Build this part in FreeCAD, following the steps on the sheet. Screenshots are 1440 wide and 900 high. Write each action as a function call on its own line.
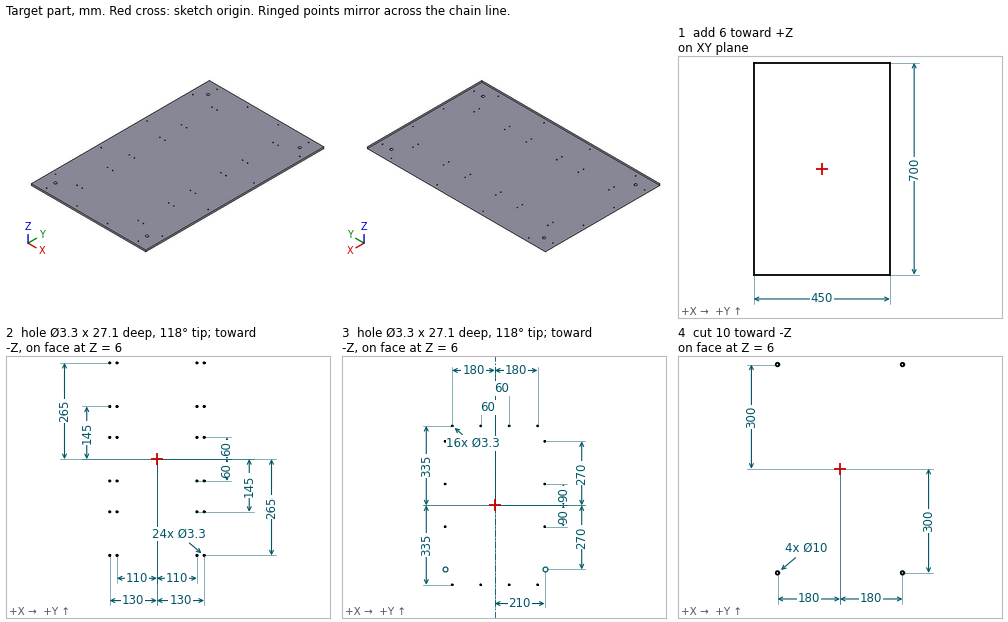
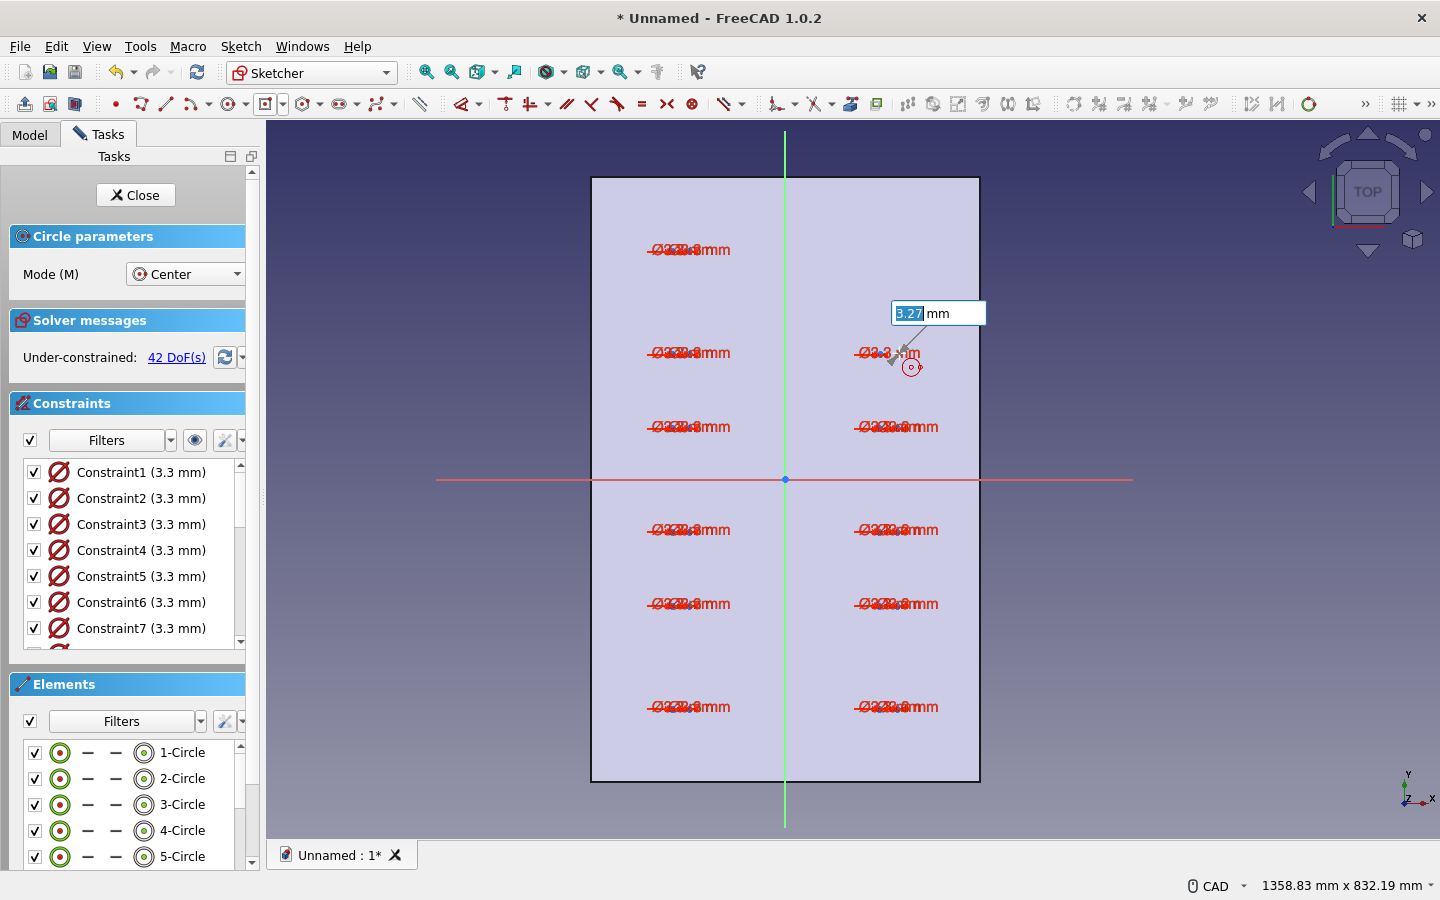
text(3.3)
key(Return)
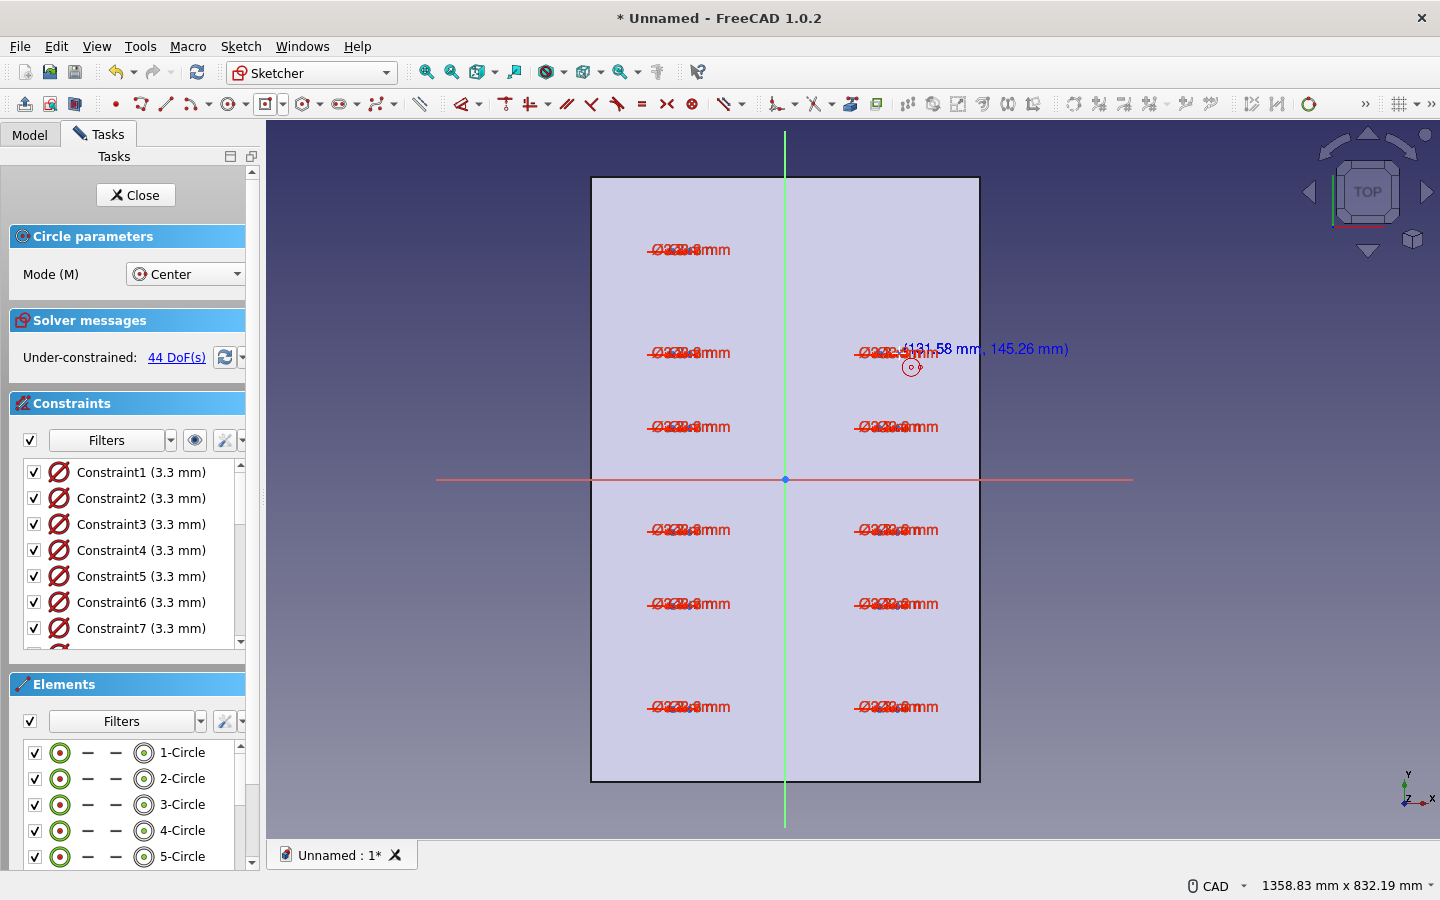
scroll(880, 251, up, 14)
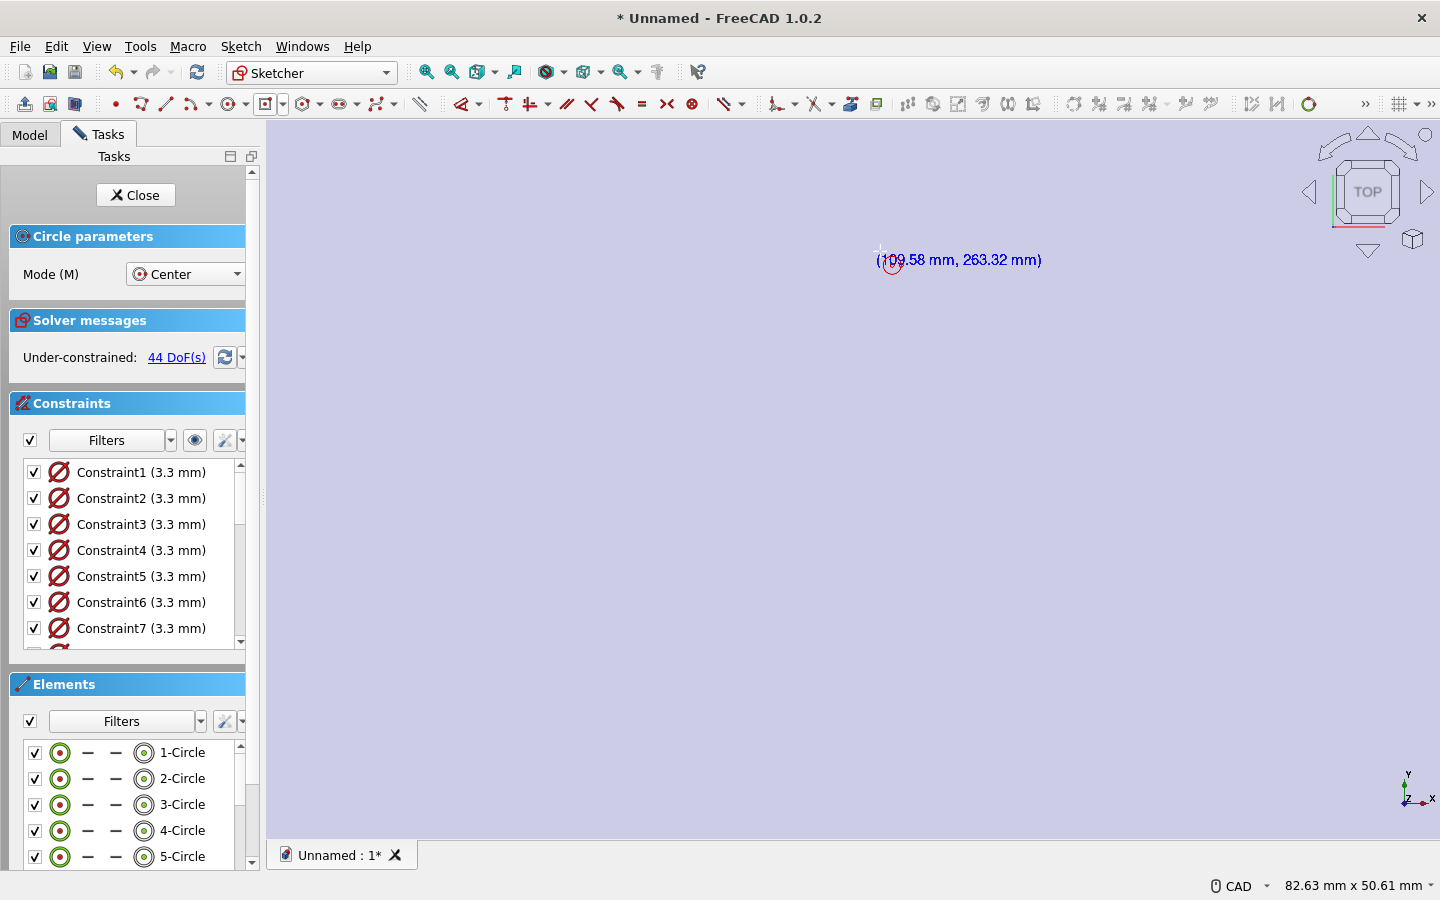
scroll(880, 251, down, 14)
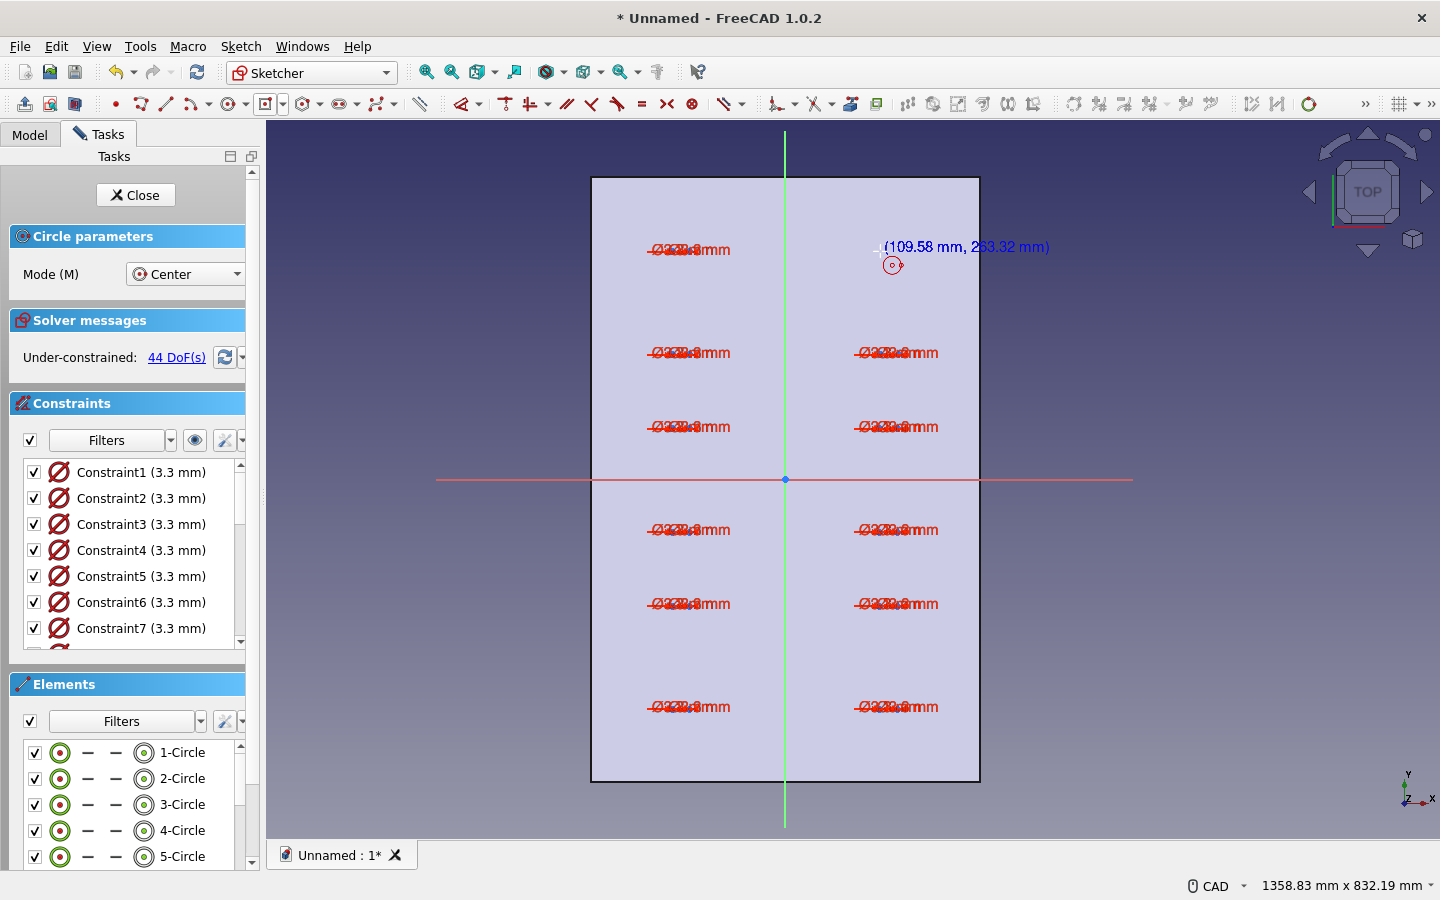
click(880, 251)
move(881, 250)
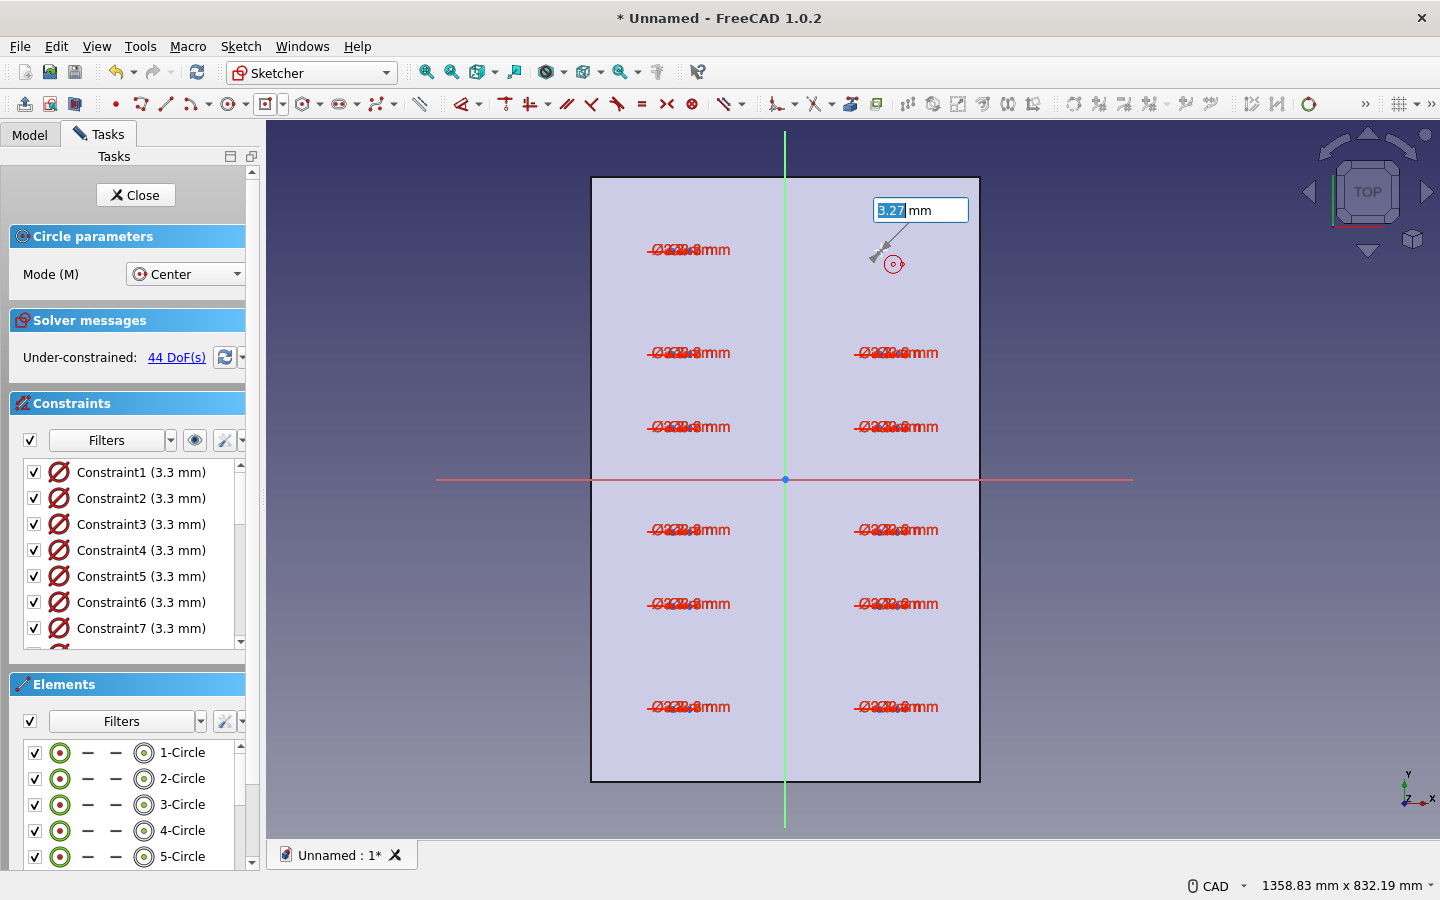
text(3.3)
key(Return)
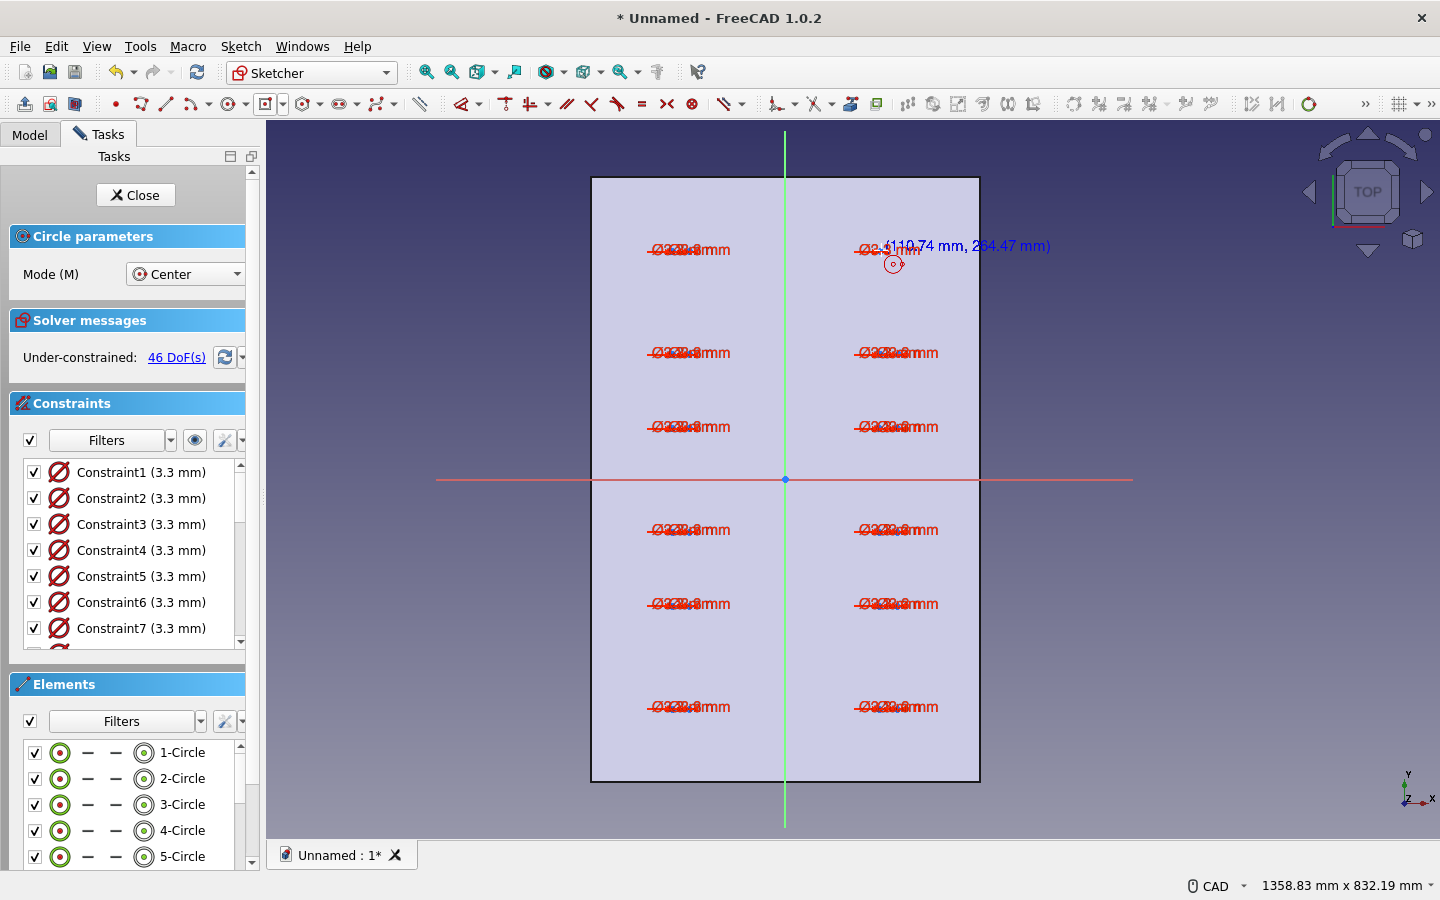
scroll(898, 251, up, 14)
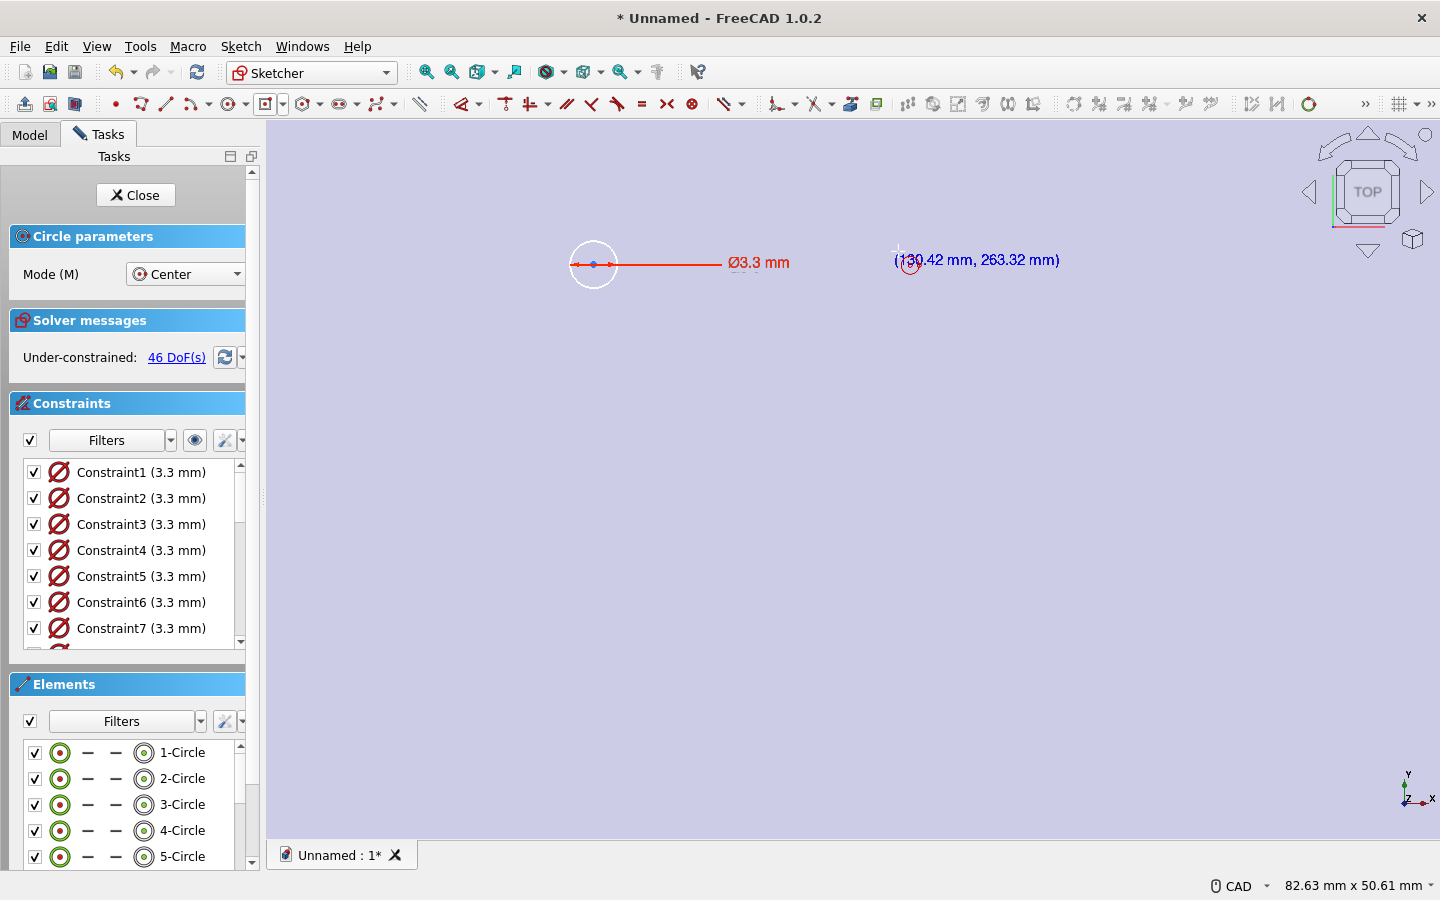
scroll(898, 251, down, 14)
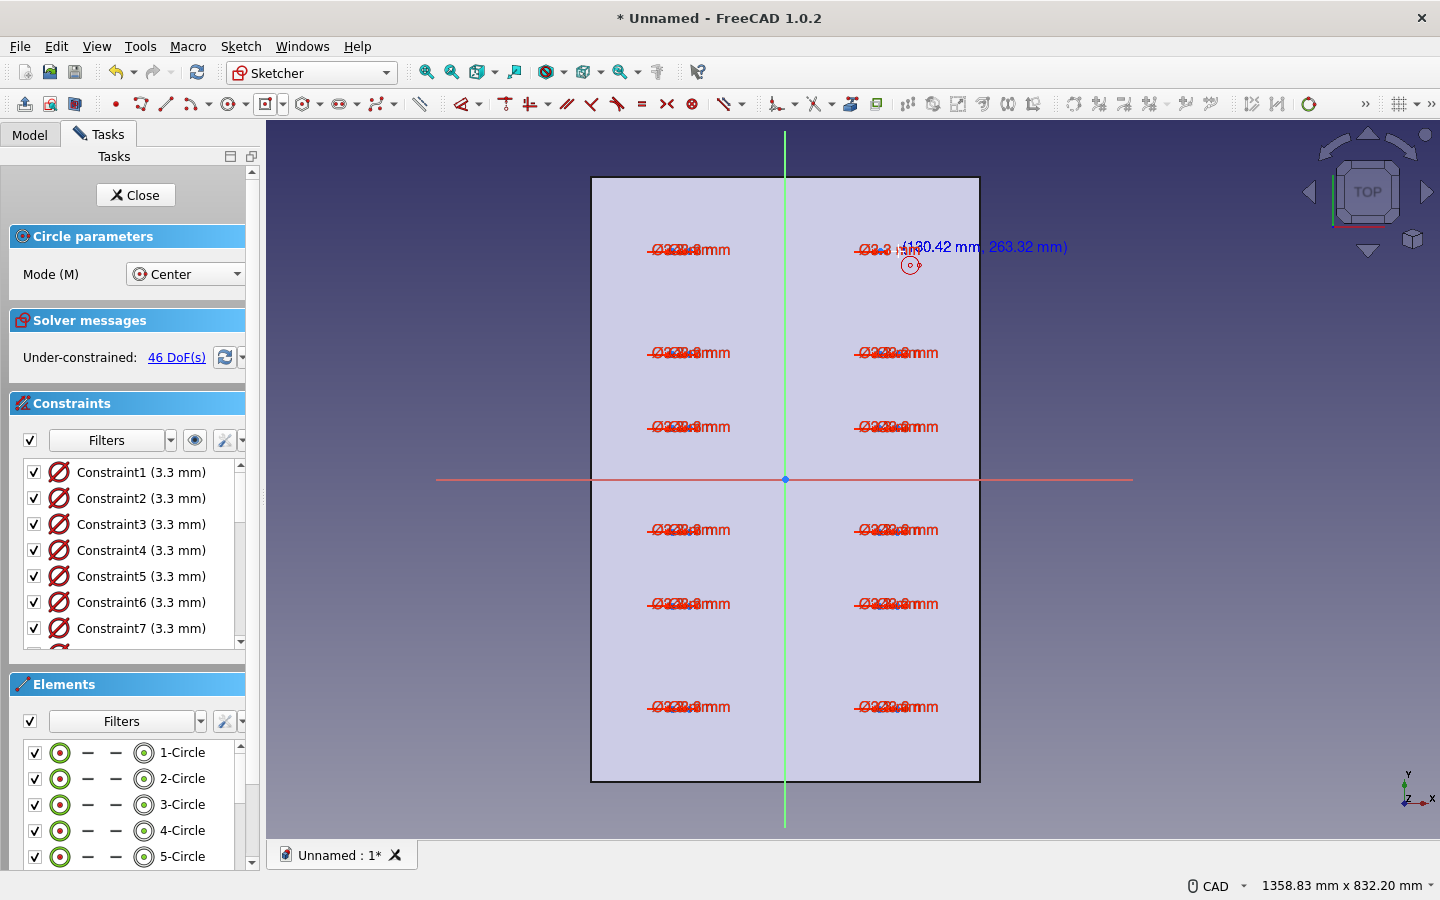
click(898, 251)
move(899, 250)